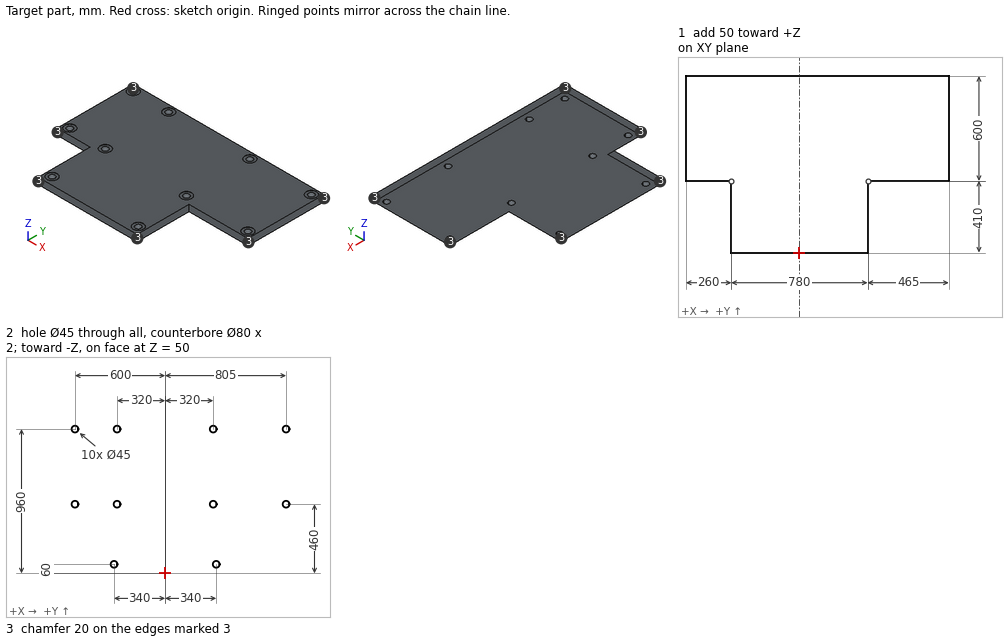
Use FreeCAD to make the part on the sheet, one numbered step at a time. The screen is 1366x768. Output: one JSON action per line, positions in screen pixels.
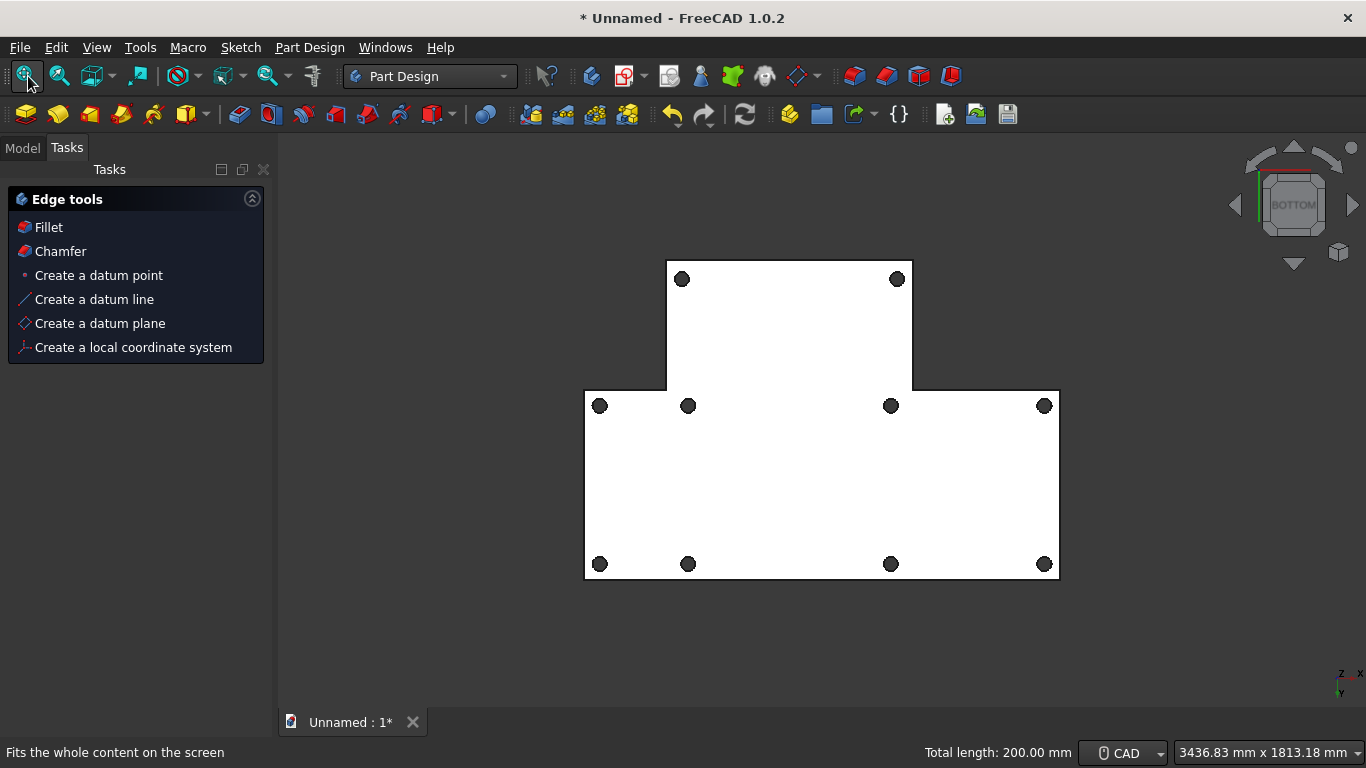
{"action": "scroll", "coordinate": [584, 579], "scroll_direction": "up", "scroll_amount": 5}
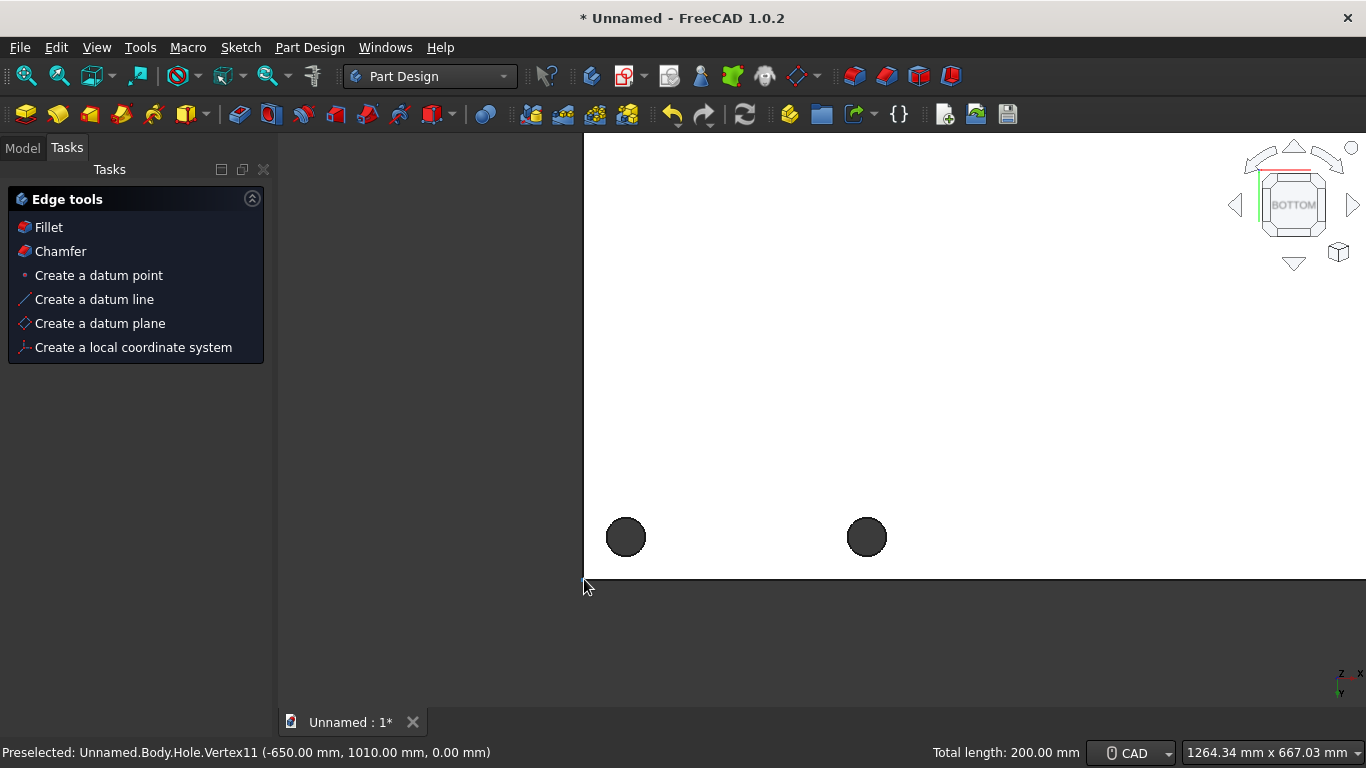
{"action": "left_click", "coordinate": [28, 76]}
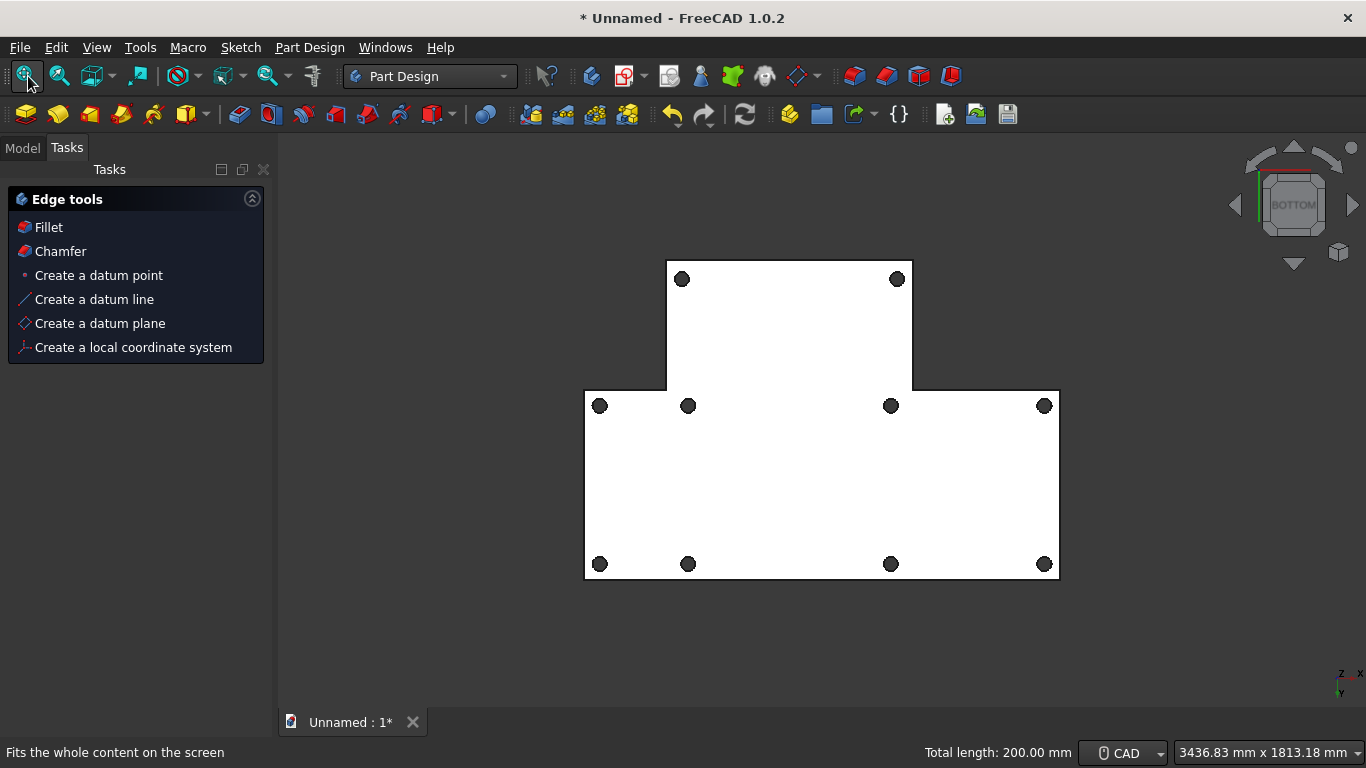
{"action": "key", "text": "4"}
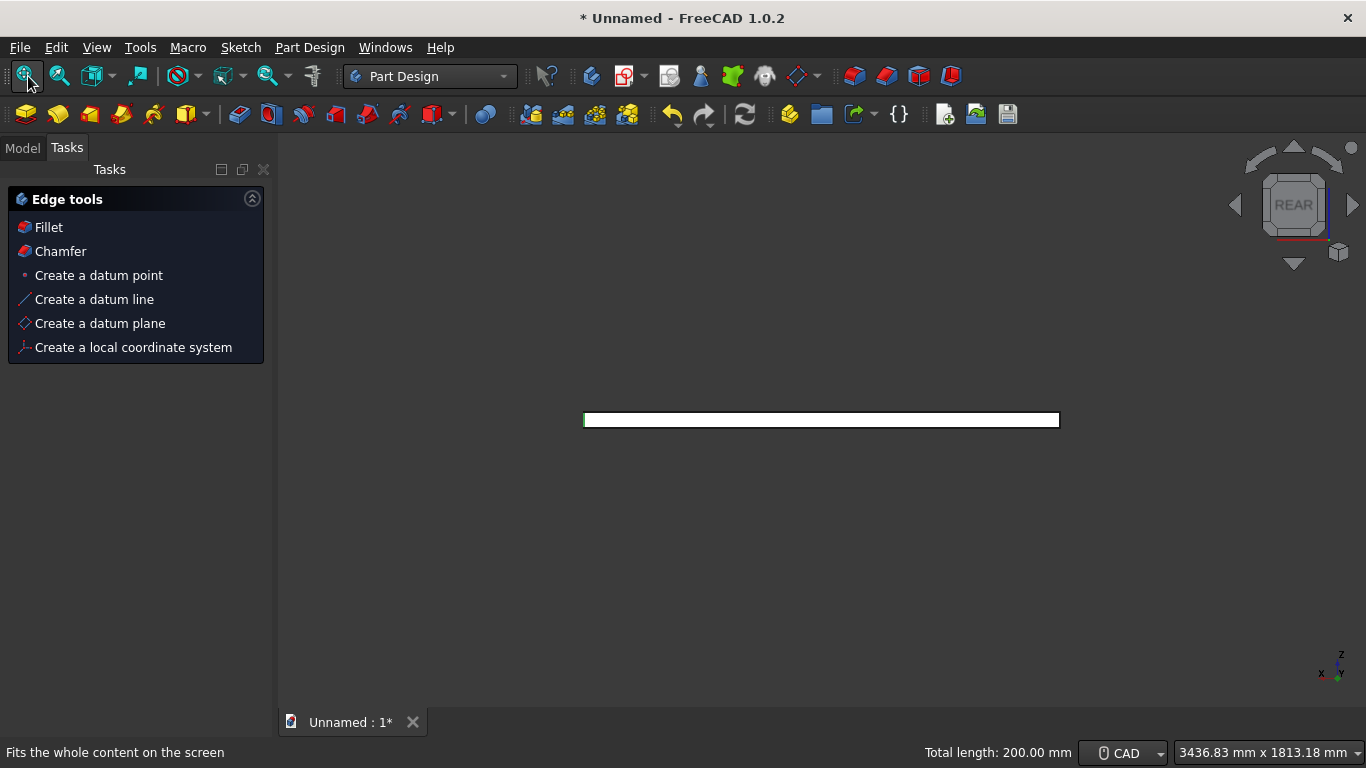
{"action": "left_click", "coordinate": [28, 76]}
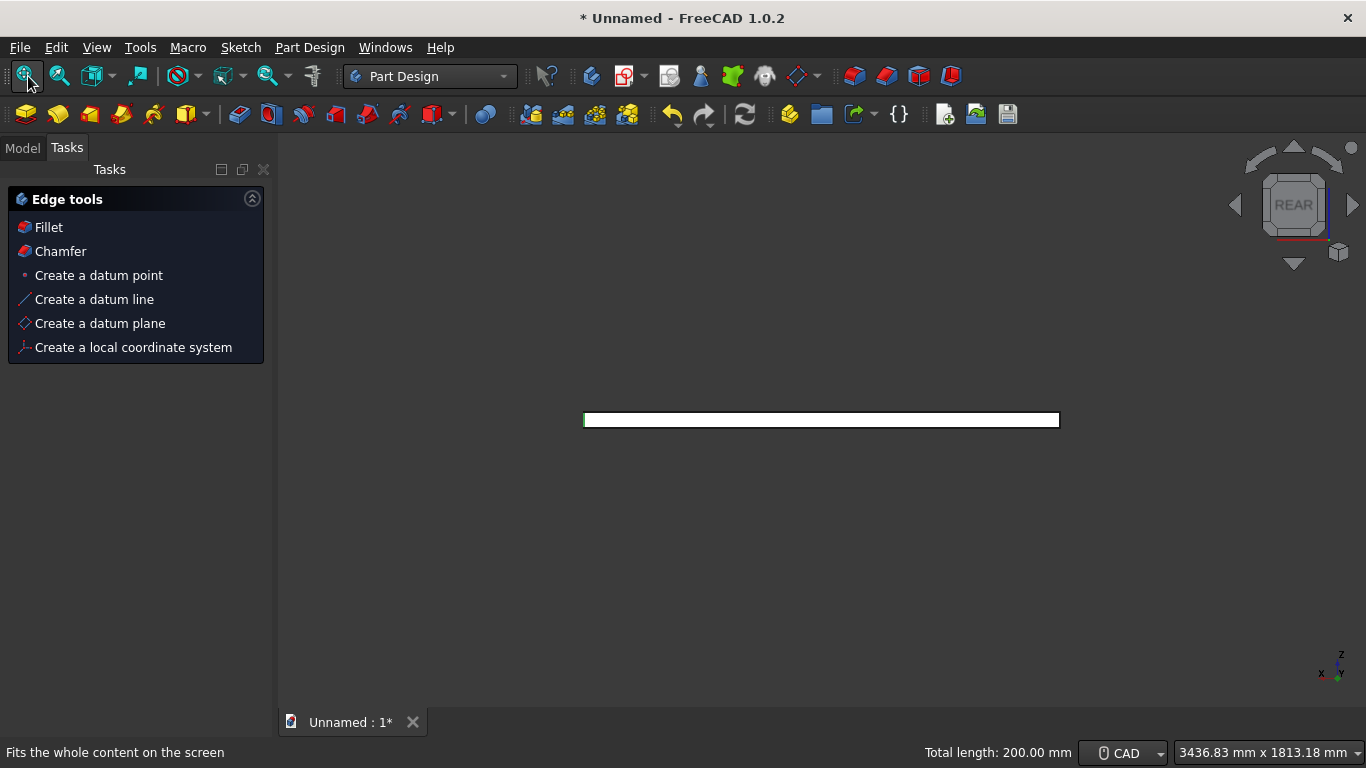
{"action": "left_click", "coordinate": [1060, 419], "text": "ctrl"}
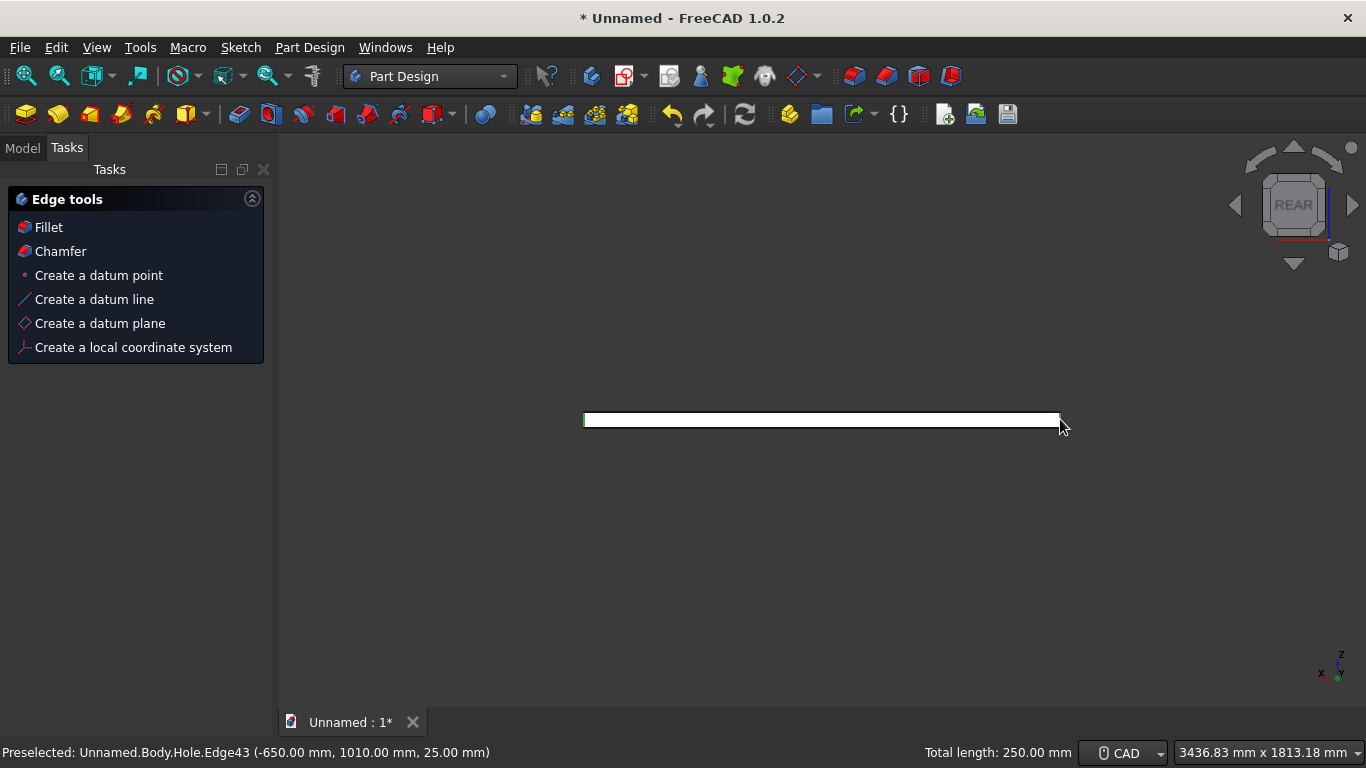
{"action": "scroll", "coordinate": [978, 419], "scroll_direction": "up", "scroll_amount": 5}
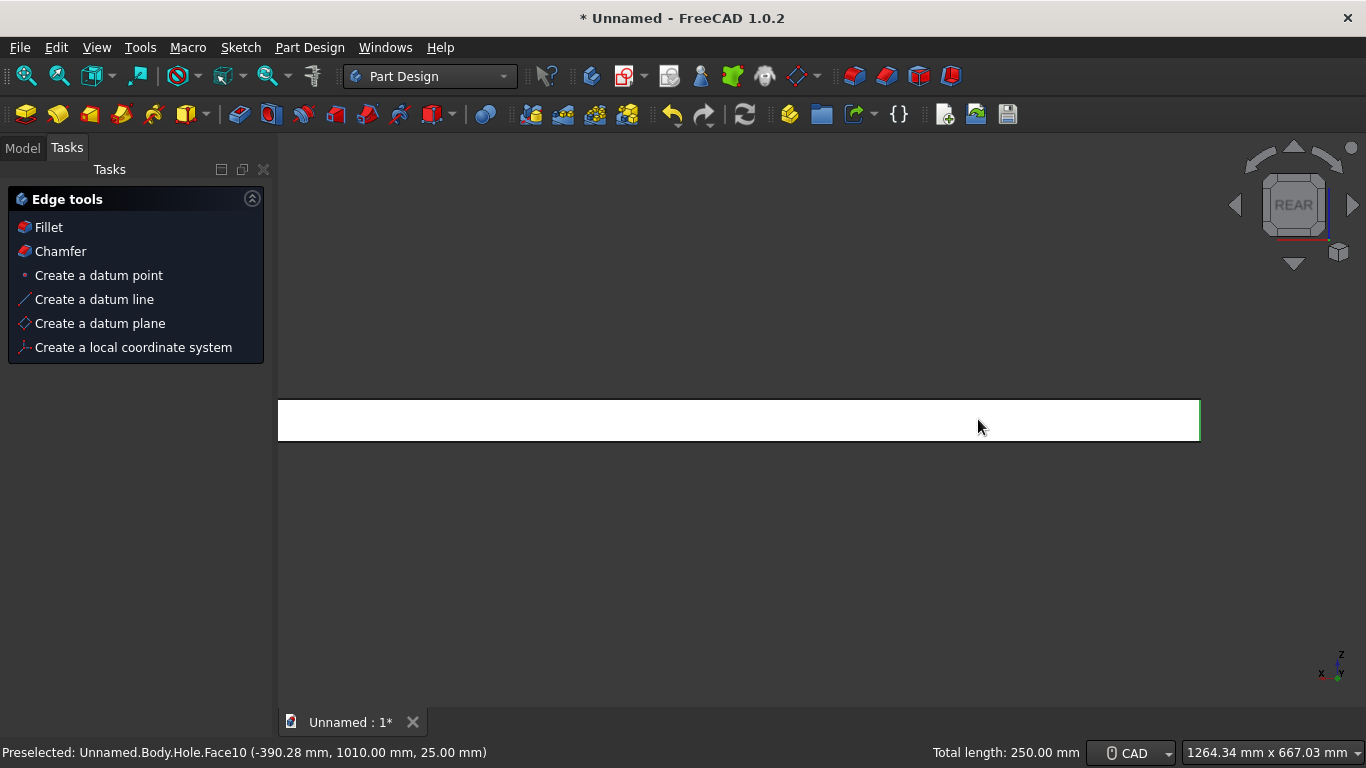
{"action": "key", "text": "v f"}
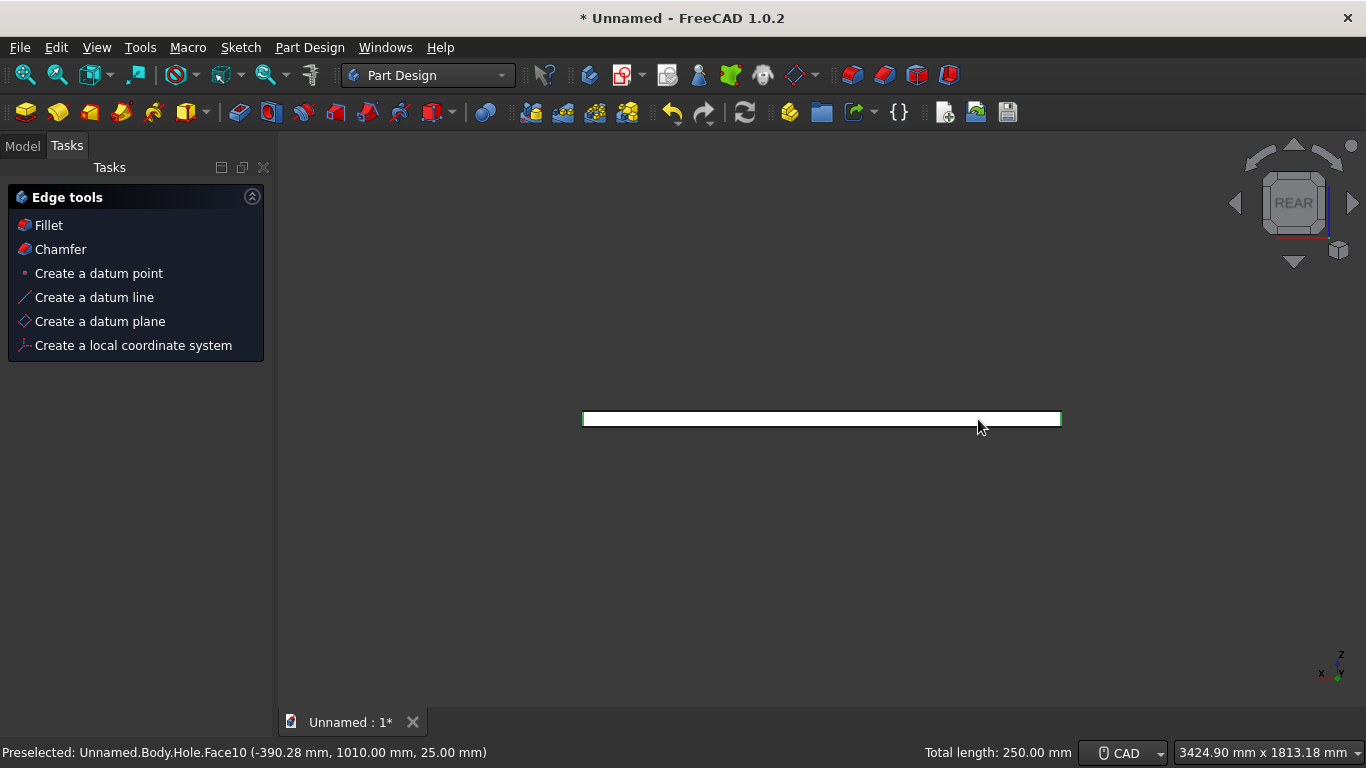
{"action": "key", "text": "6"}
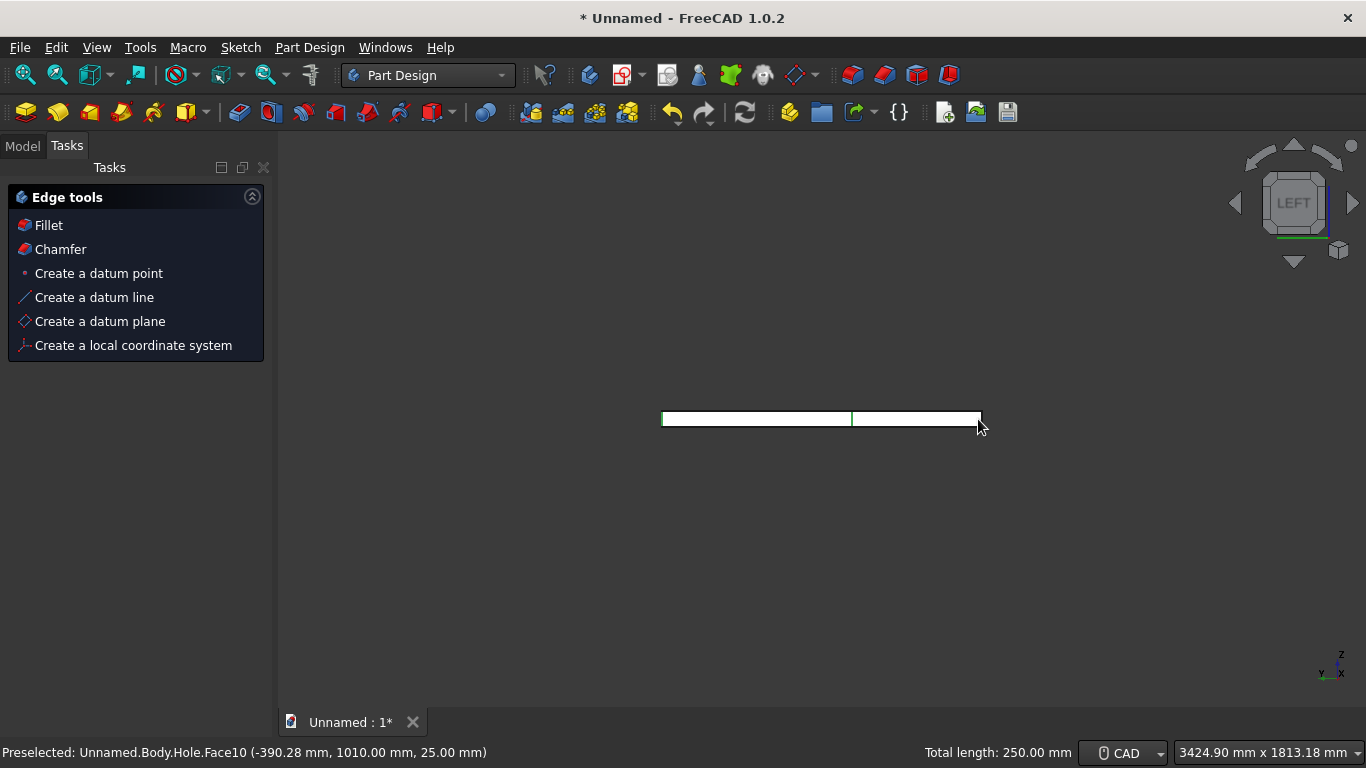
{"action": "left_click", "coordinate": [26, 76]}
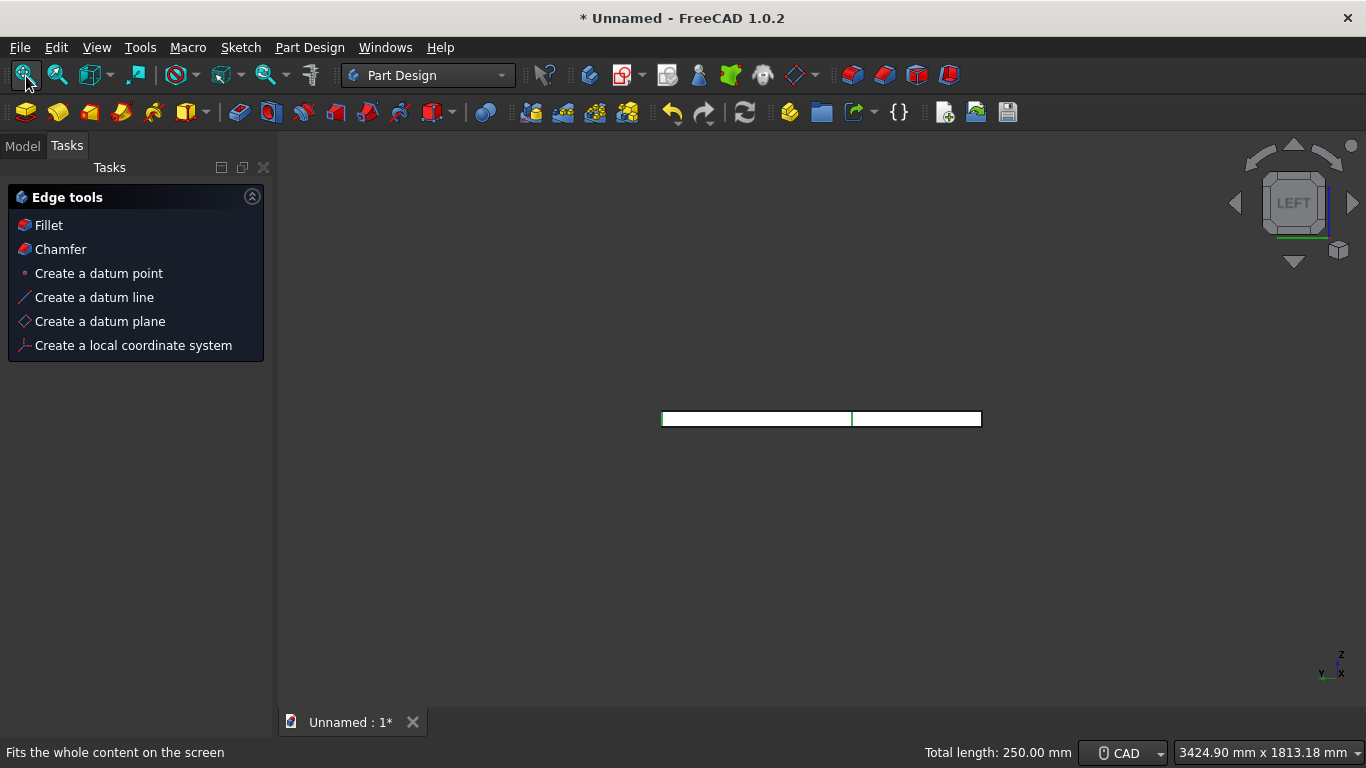
{"action": "left_click", "coordinate": [982, 418], "text": "ctrl"}